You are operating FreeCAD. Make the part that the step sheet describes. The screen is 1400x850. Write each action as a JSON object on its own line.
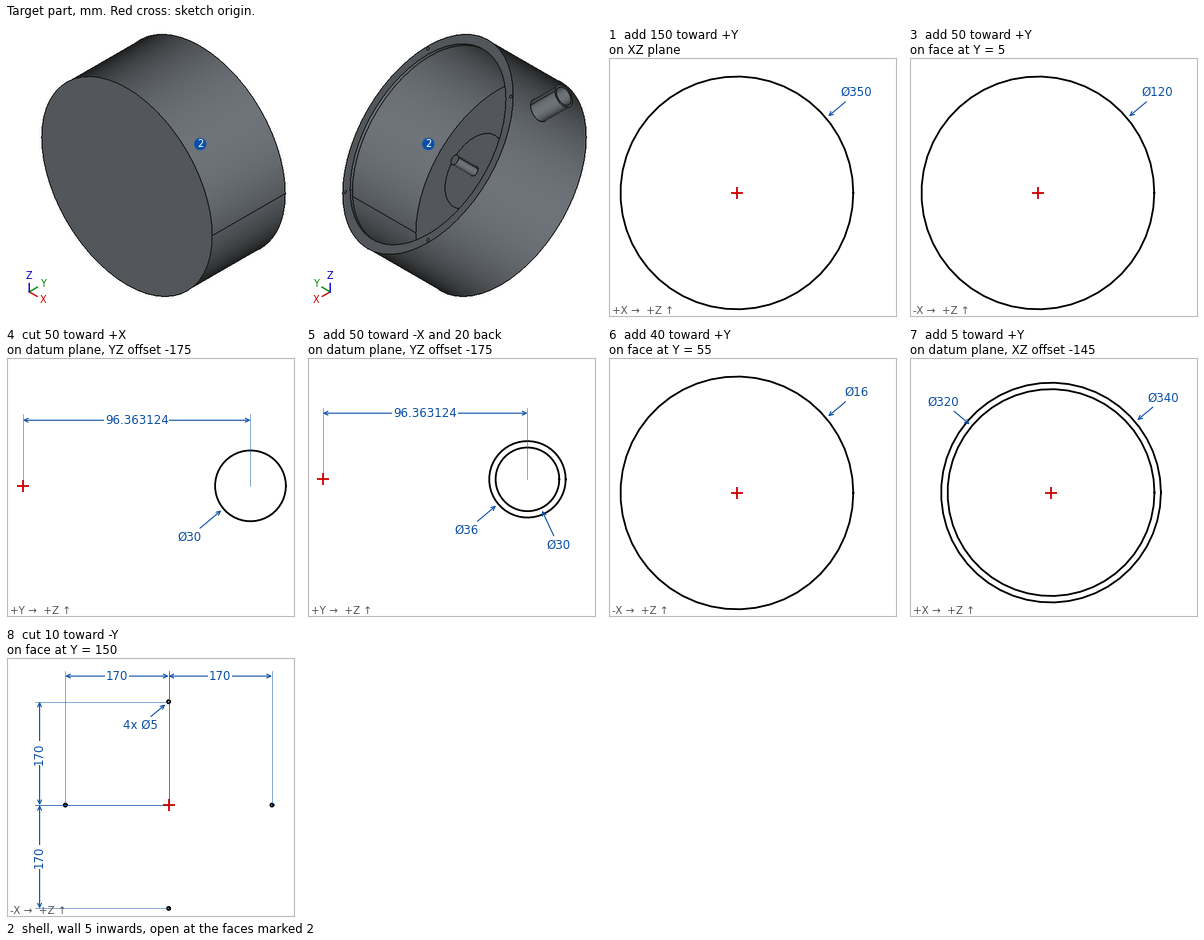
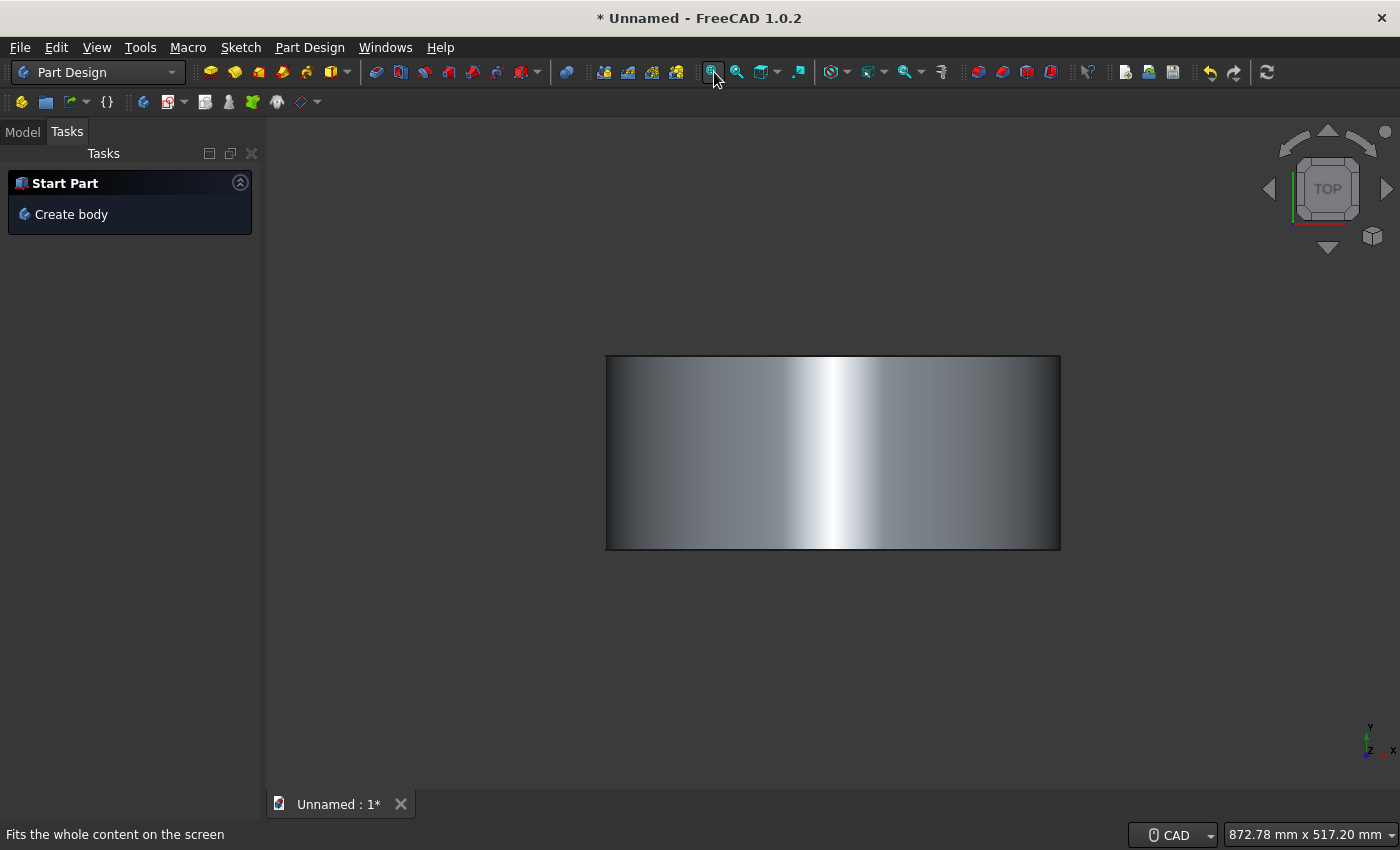
{"action": "left_click", "coordinate": [714, 72]}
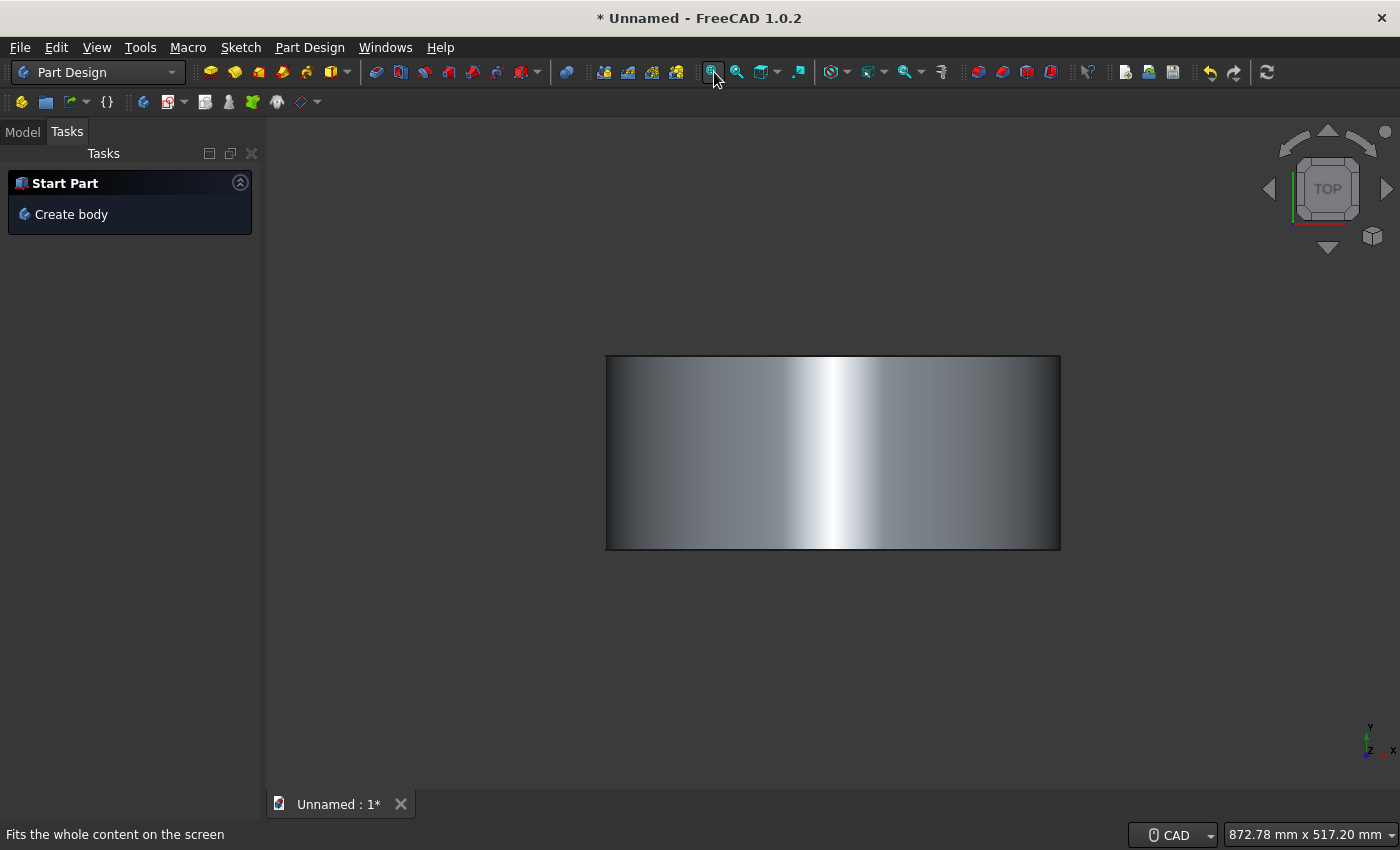
{"action": "key", "text": "1"}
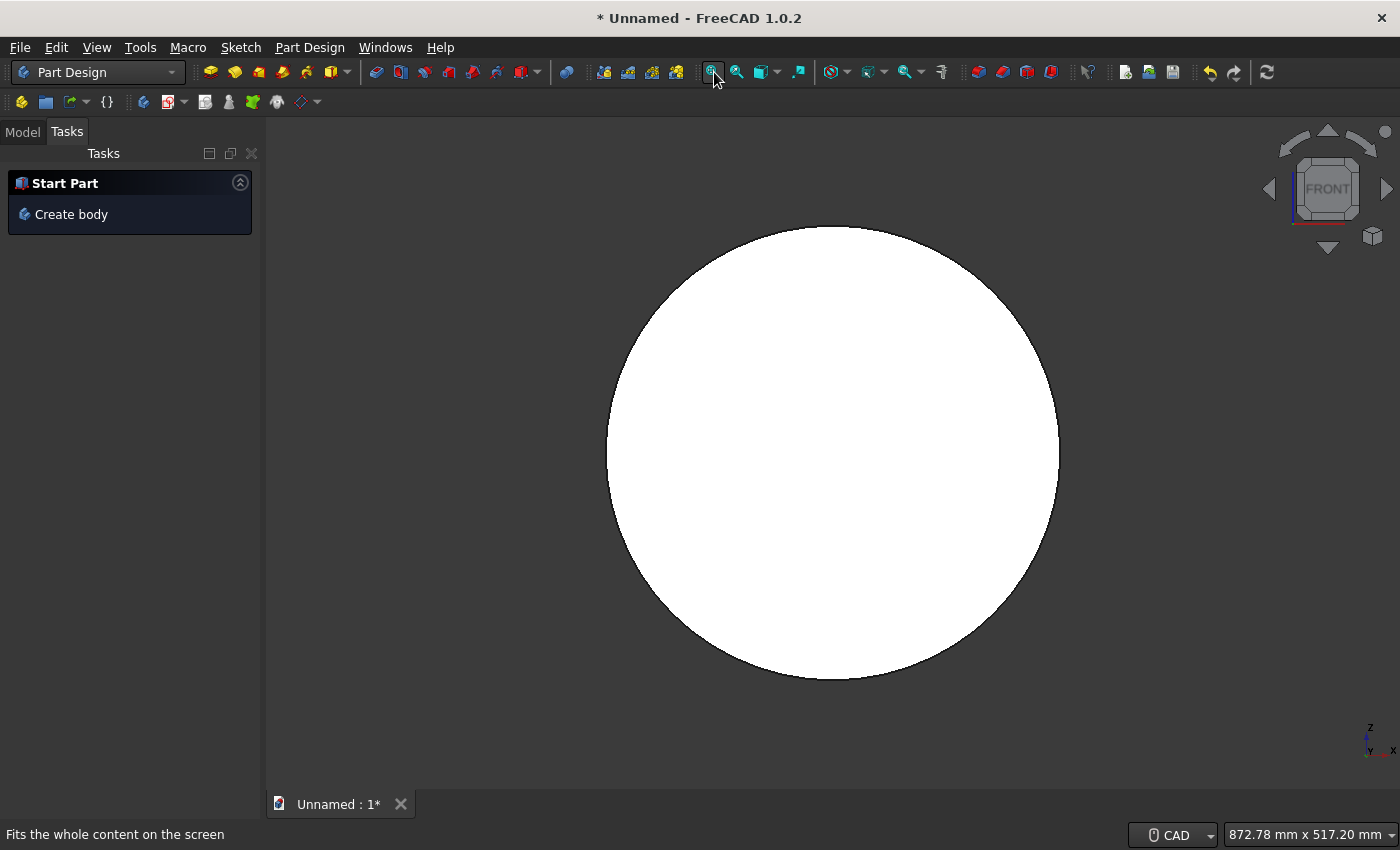
{"action": "key", "text": "3"}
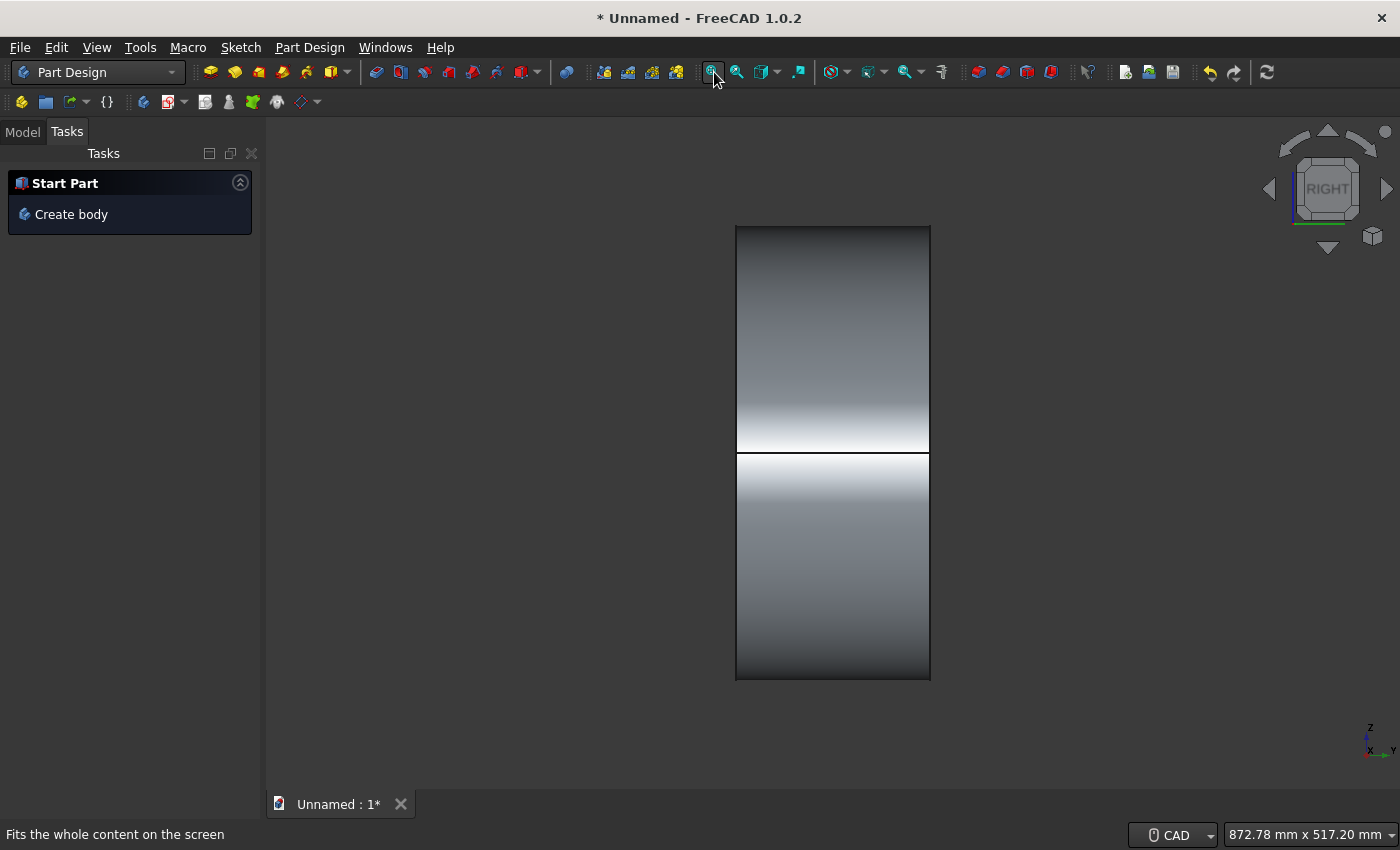
{"action": "key", "text": "5"}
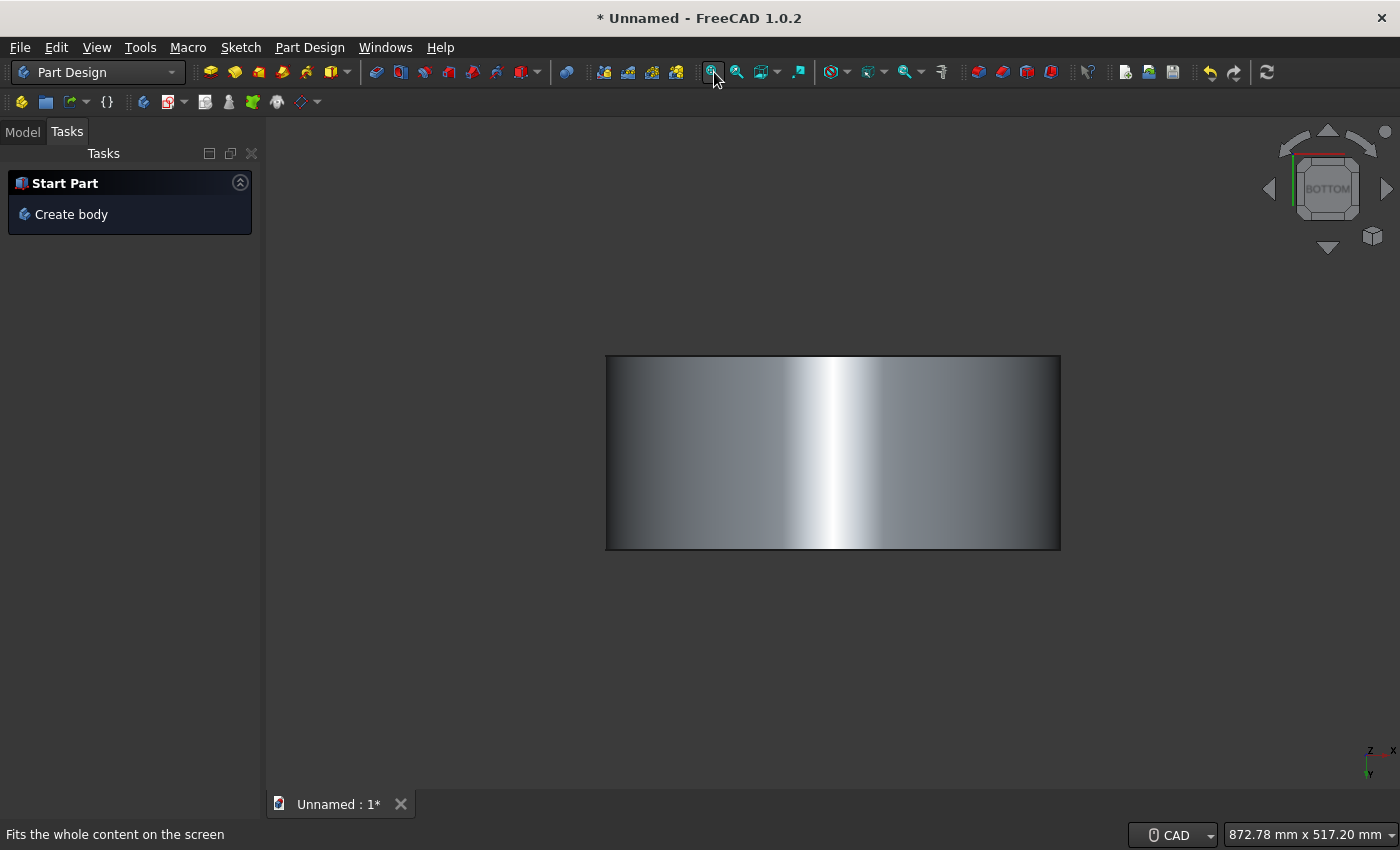
{"action": "left_click", "coordinate": [714, 72]}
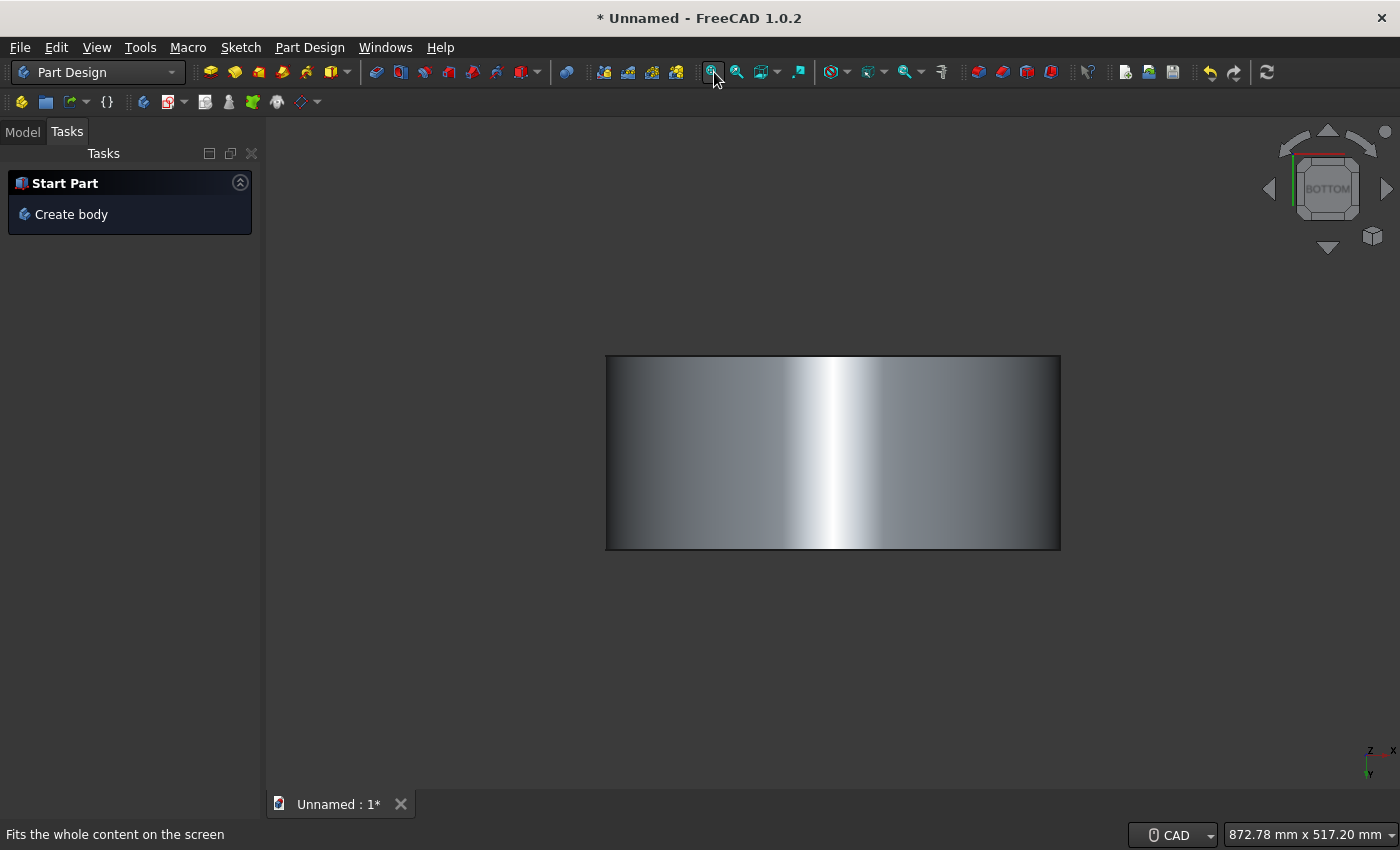
{"action": "key", "text": "4"}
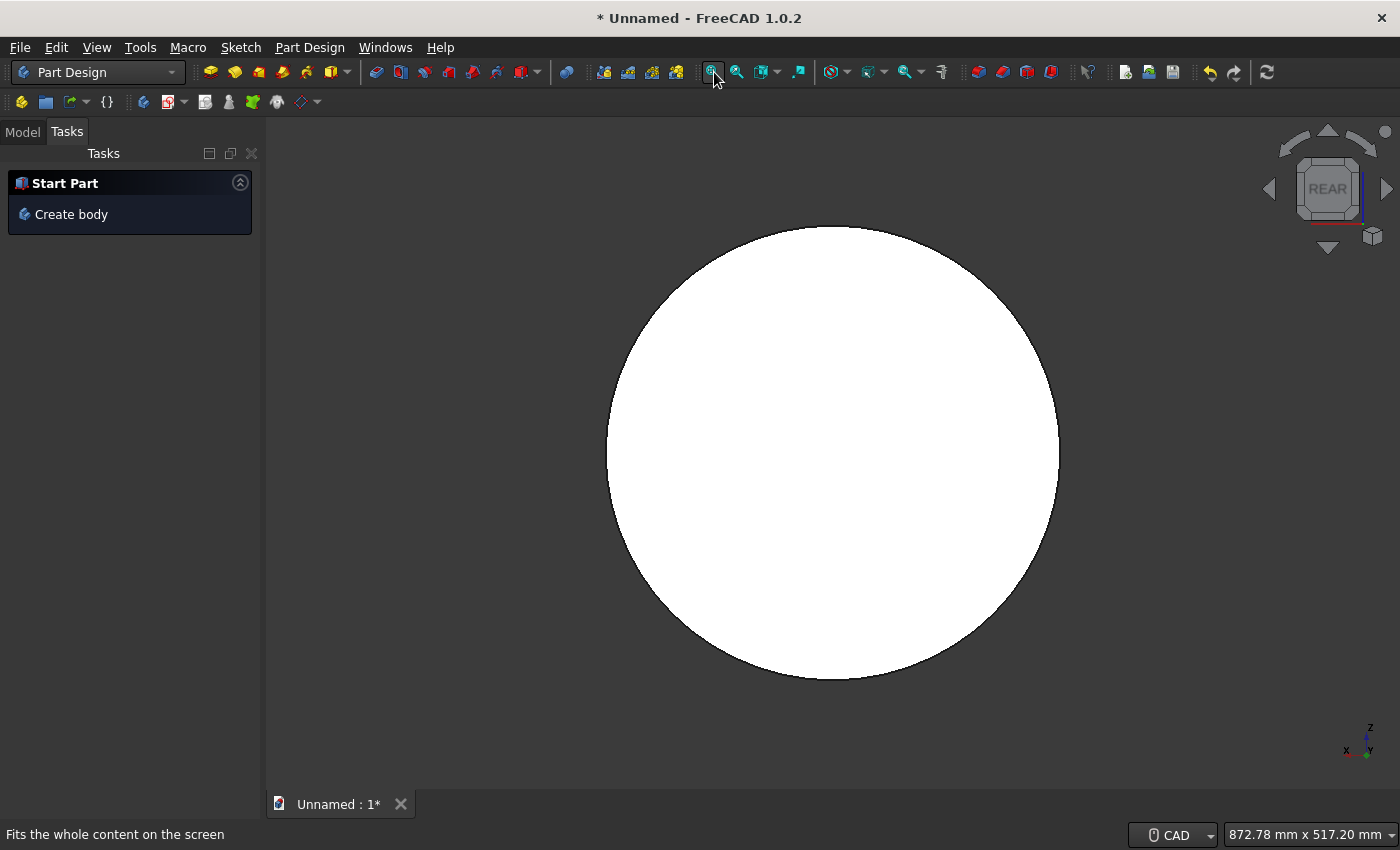
{"action": "left_click", "coordinate": [833, 452]}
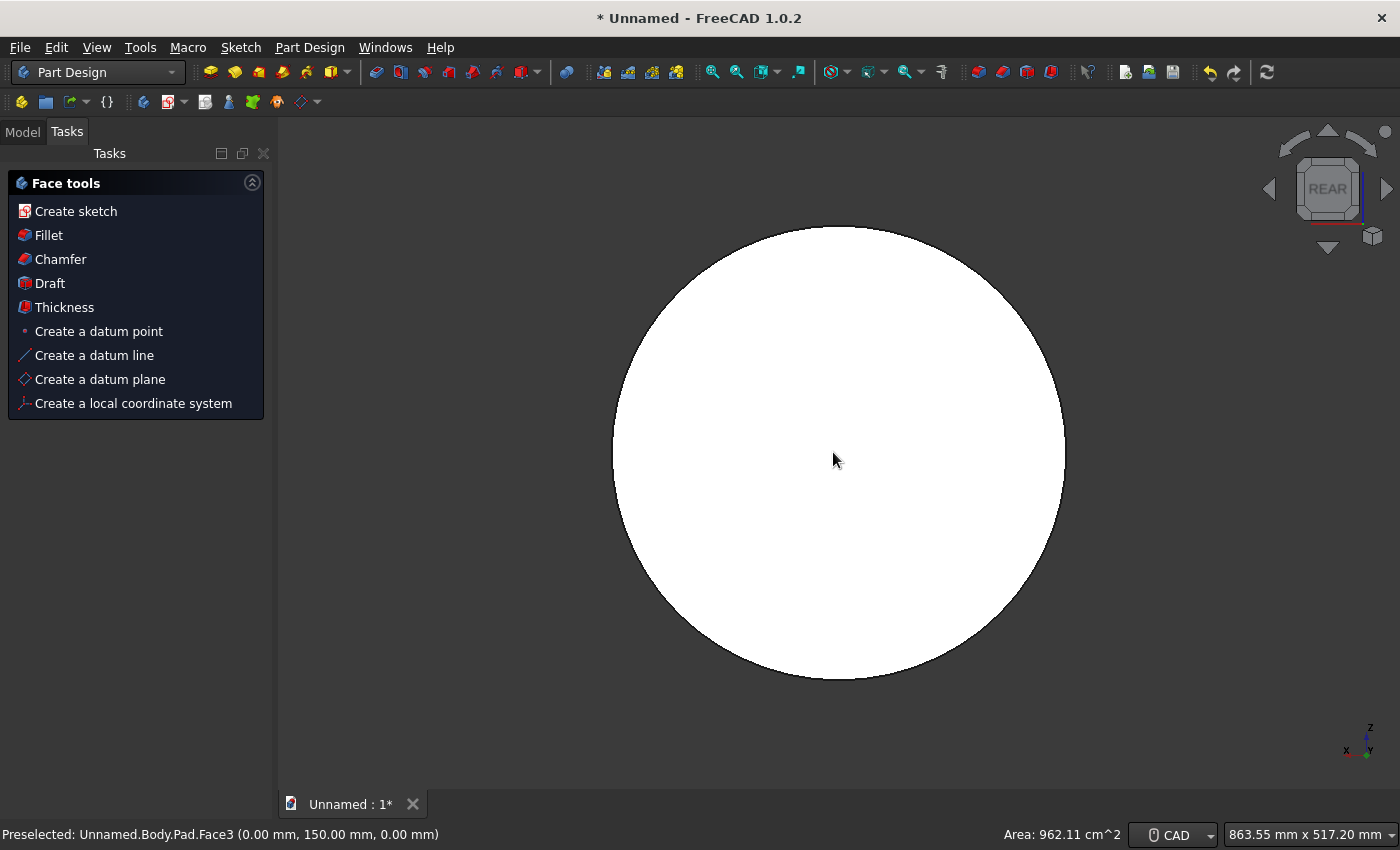
{"action": "left_click", "coordinate": [1052, 72]}